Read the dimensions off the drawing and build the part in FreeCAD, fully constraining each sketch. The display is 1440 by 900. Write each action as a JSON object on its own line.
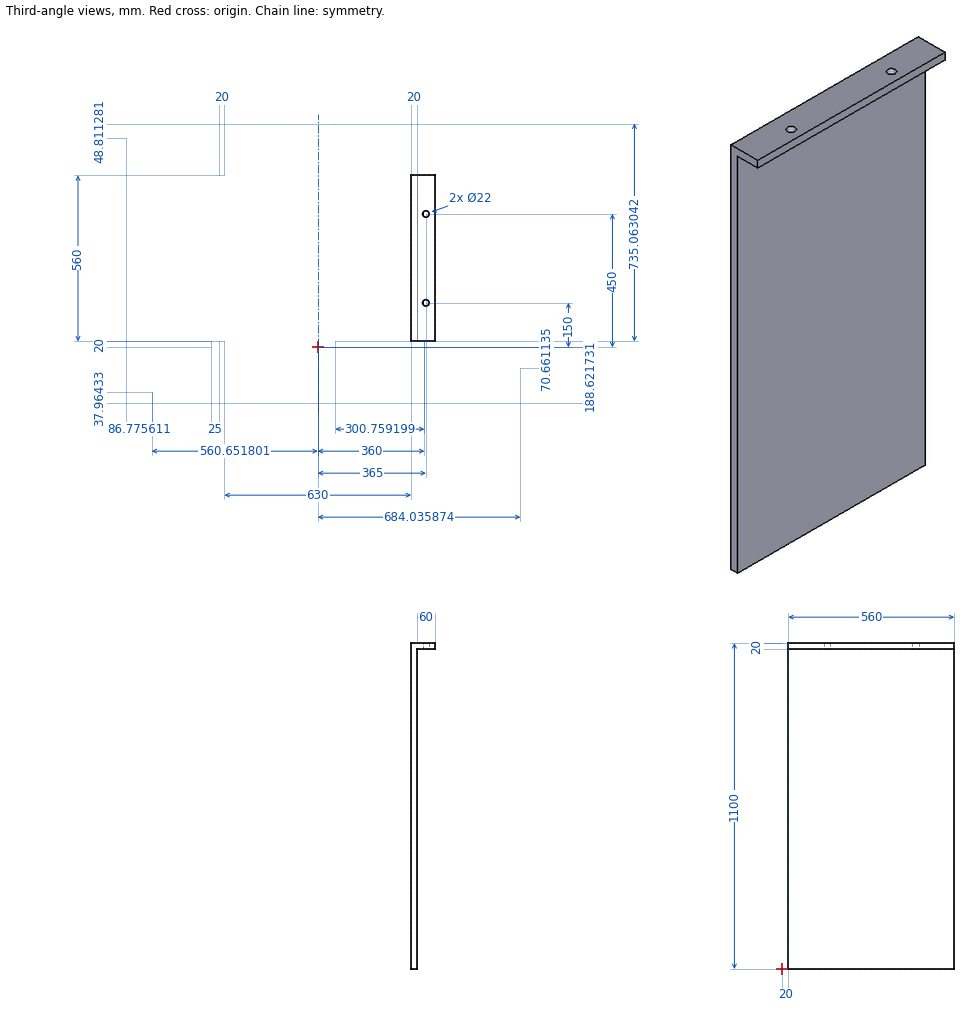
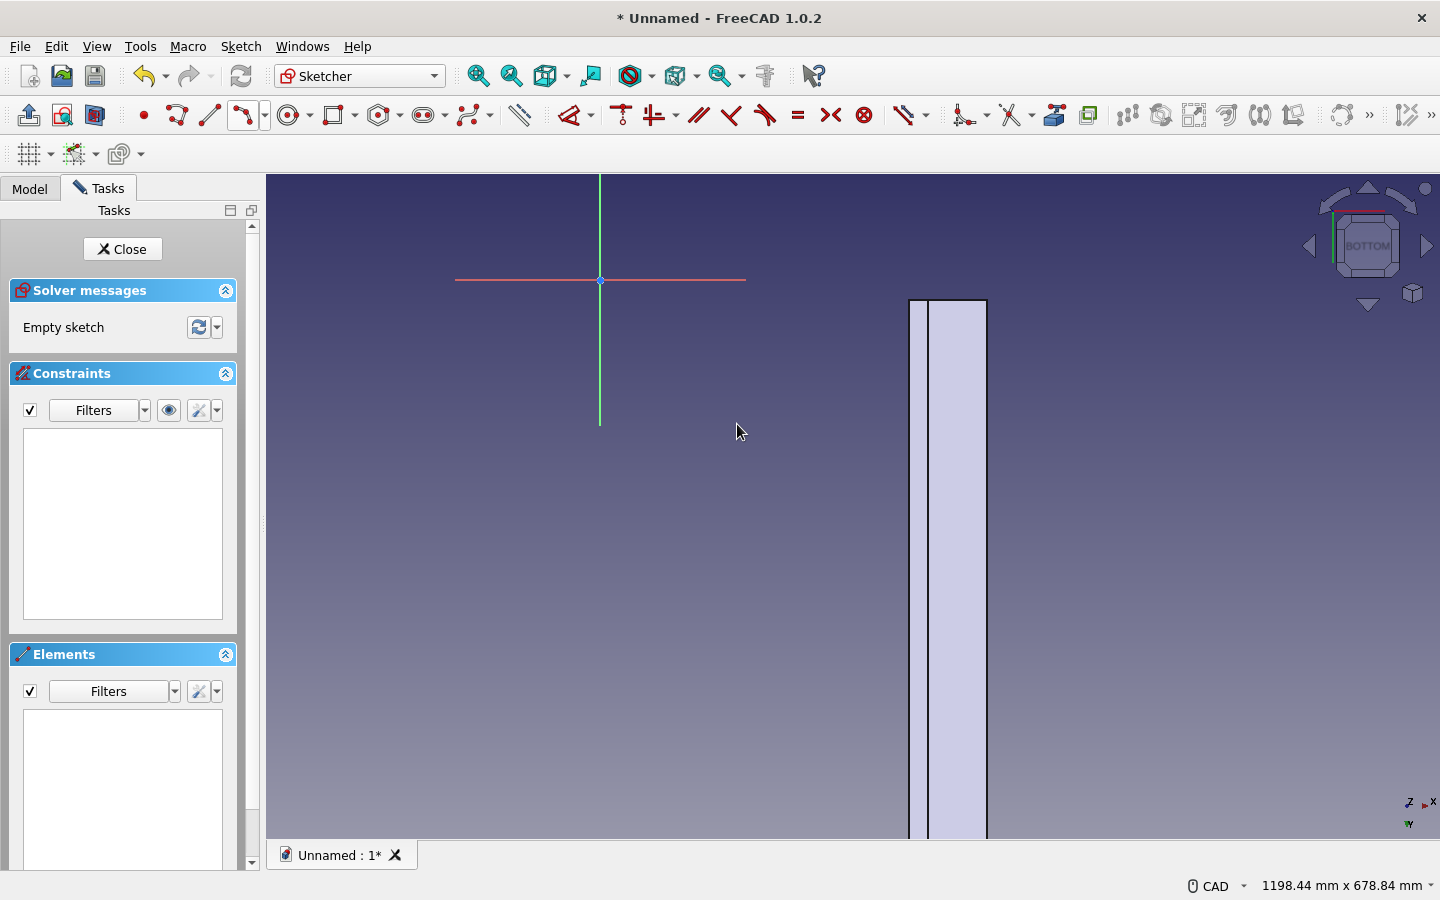
{"action": "key", "text": "g c"}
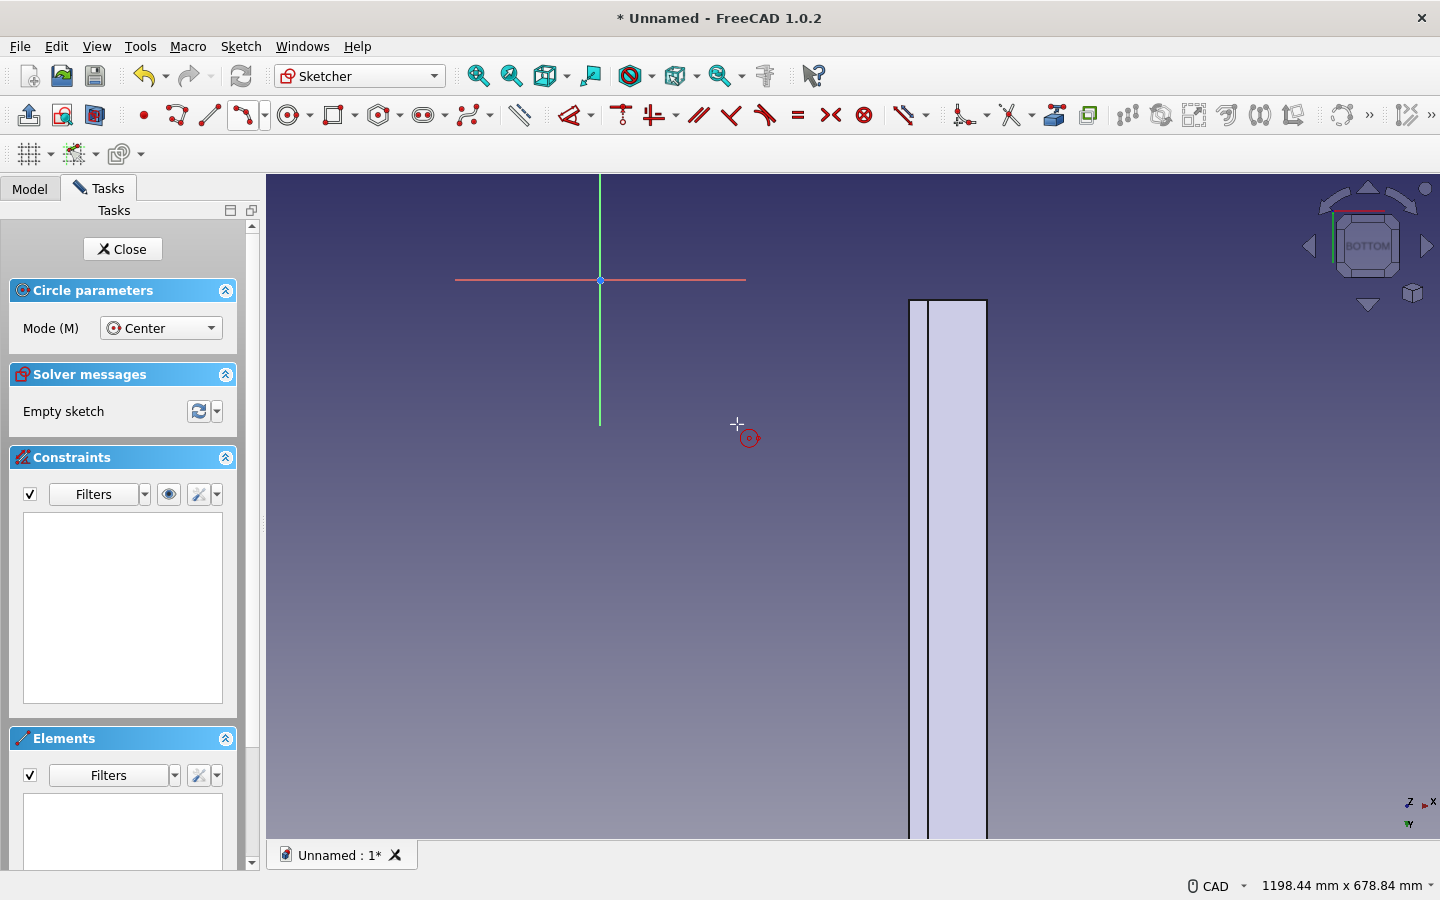
{"action": "scroll", "coordinate": [958, 721], "scroll_direction": "up", "scroll_amount": 4}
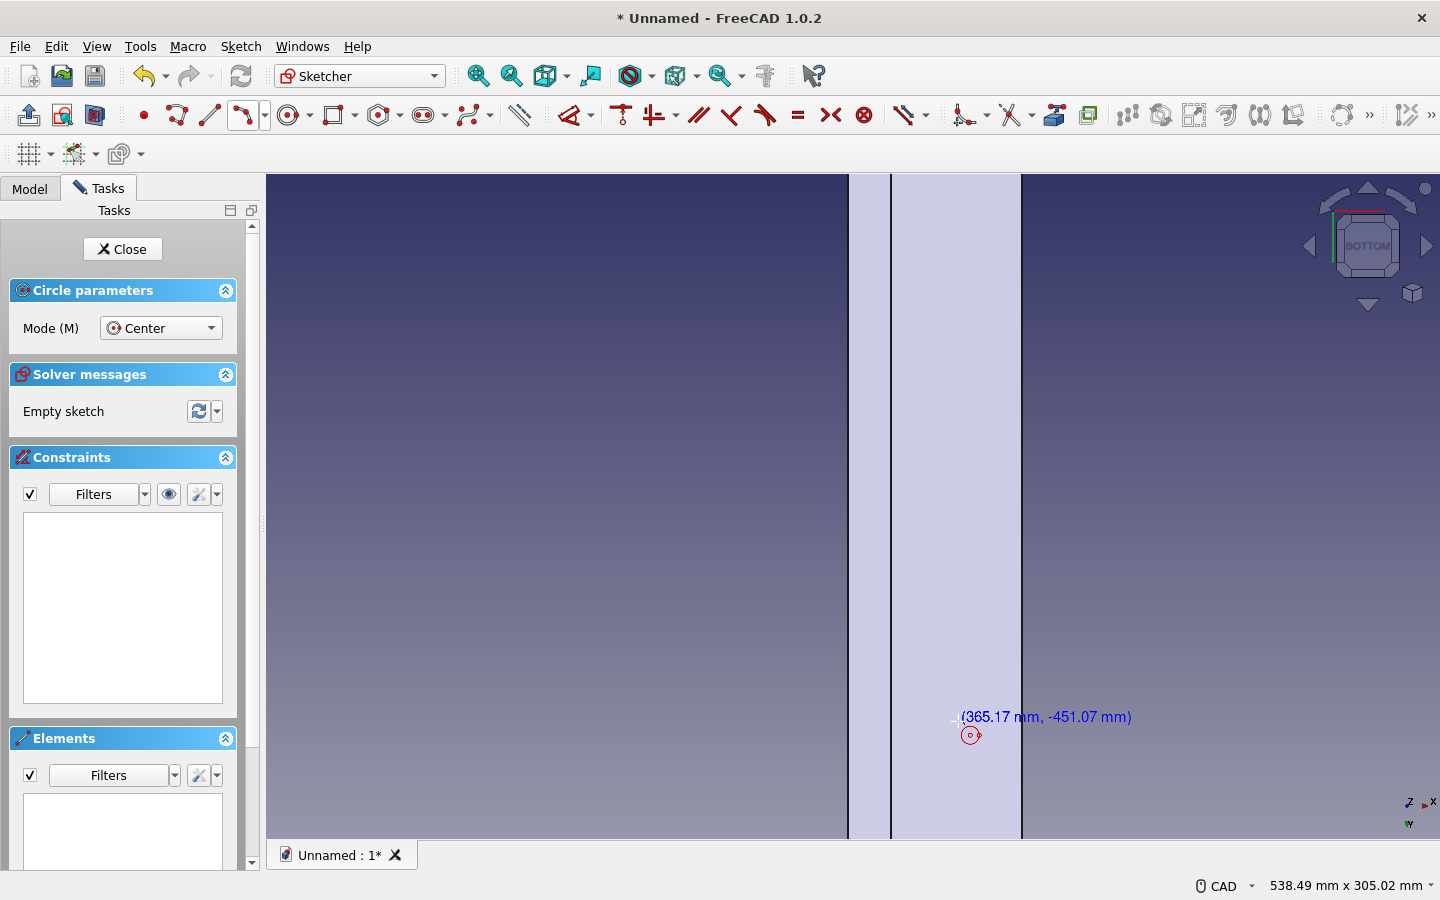
{"action": "left_click", "coordinate": [957, 720]}
{"action": "left_click", "coordinate": [974, 703]}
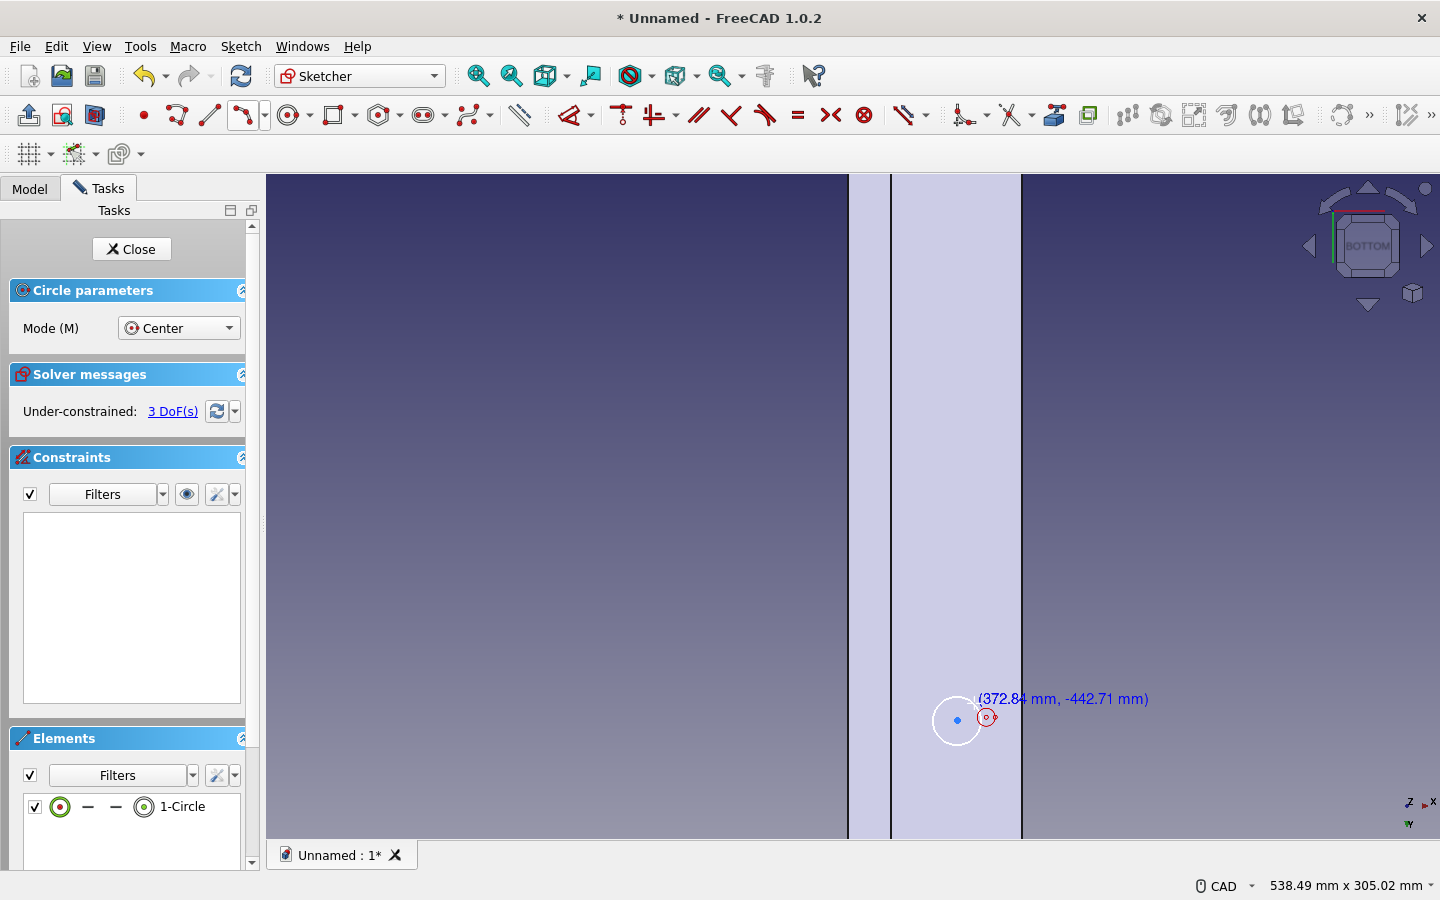
{"action": "scroll", "coordinate": [959, 723], "scroll_direction": "down", "scroll_amount": 4}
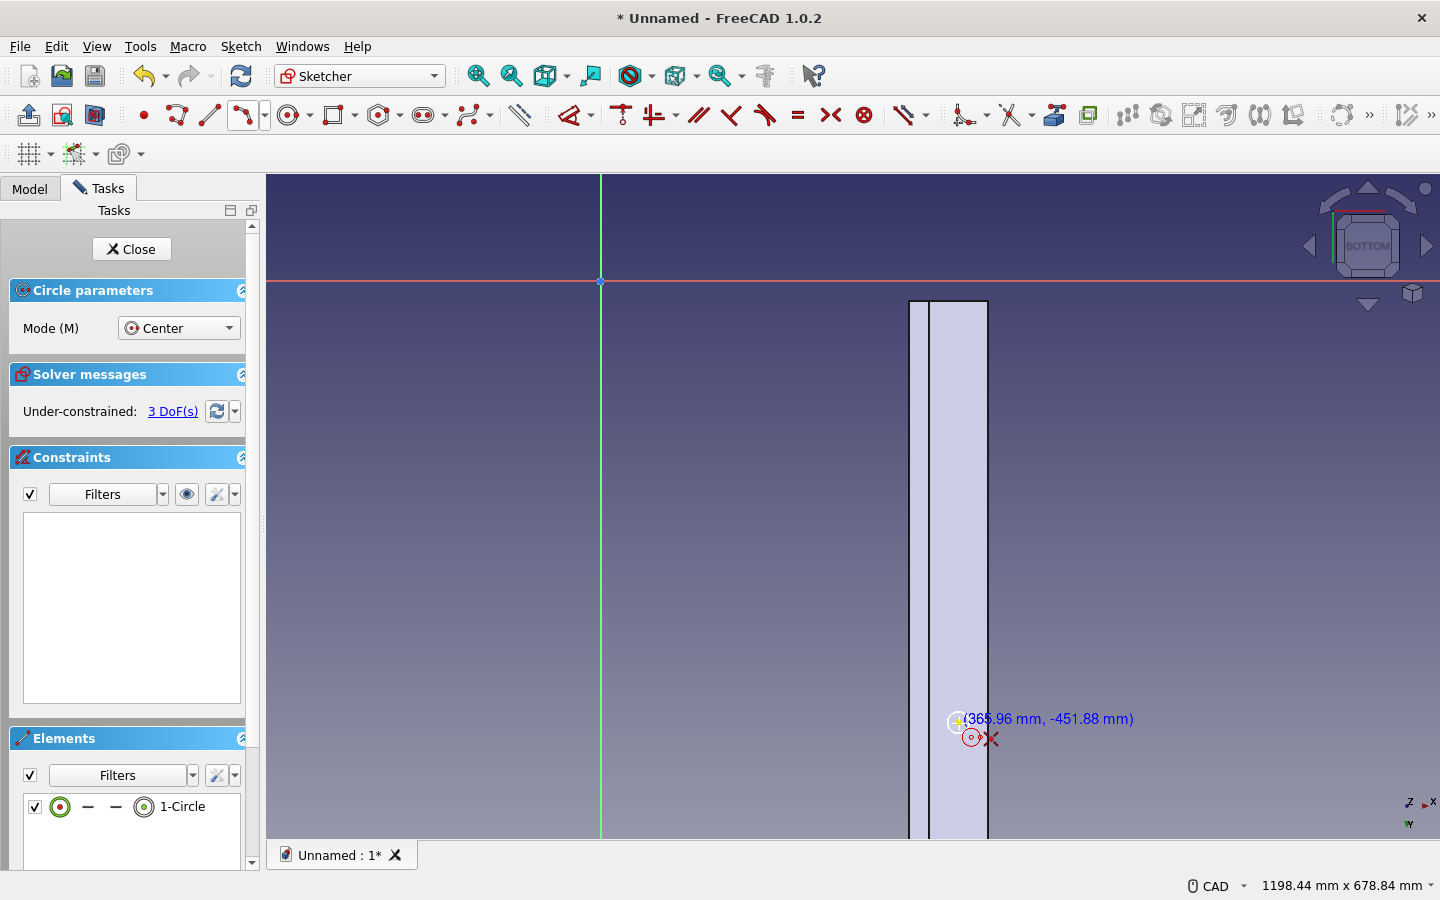
{"action": "scroll", "coordinate": [958, 428], "scroll_direction": "up", "scroll_amount": 4}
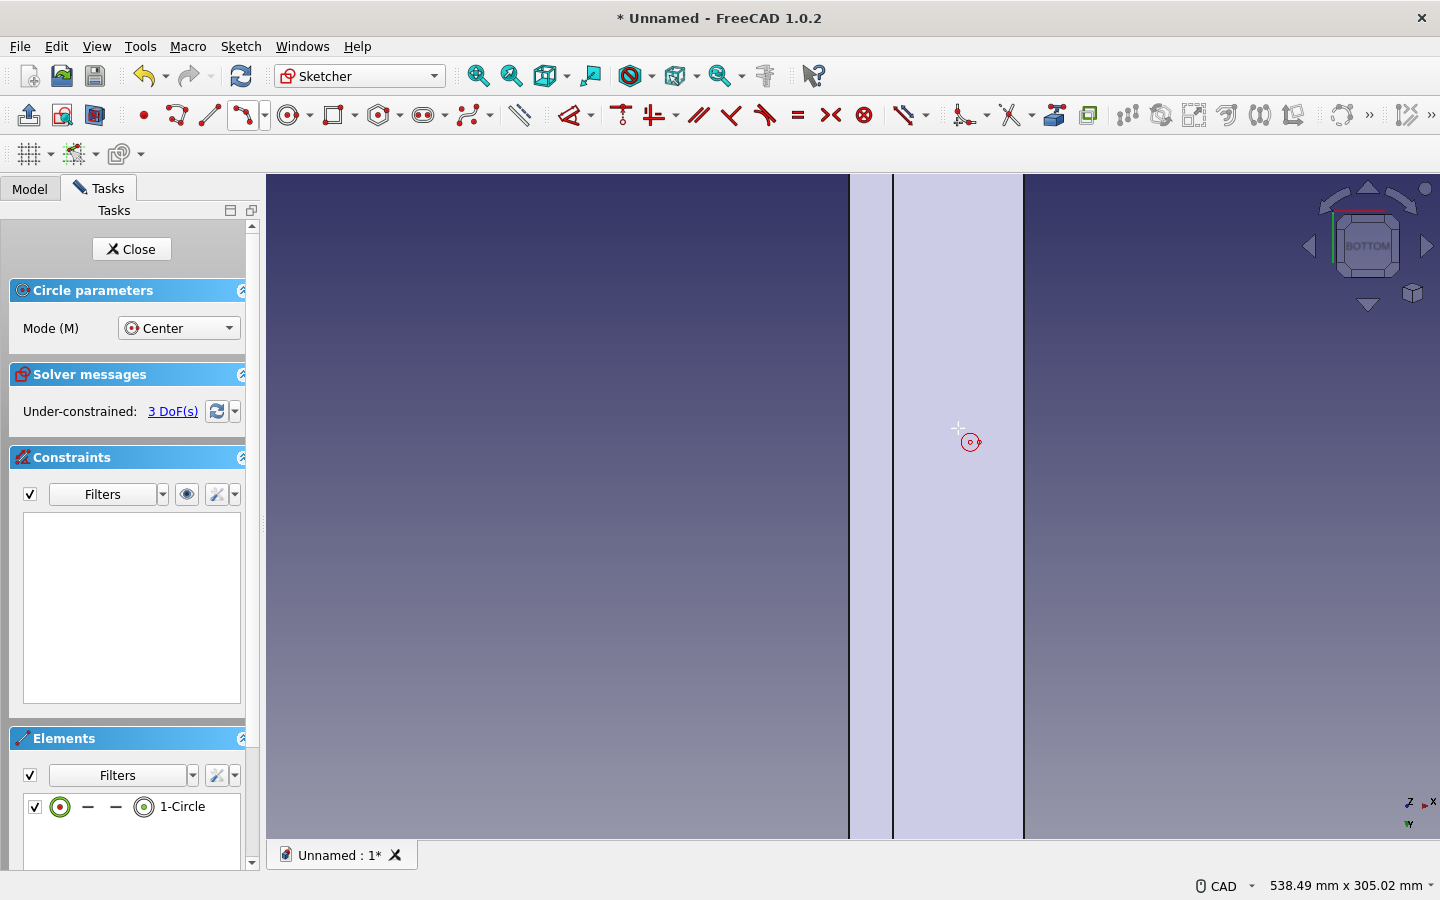
{"action": "left_click", "coordinate": [958, 428]}
{"action": "left_click", "coordinate": [975, 411]}
{"action": "key", "text": "Escape"}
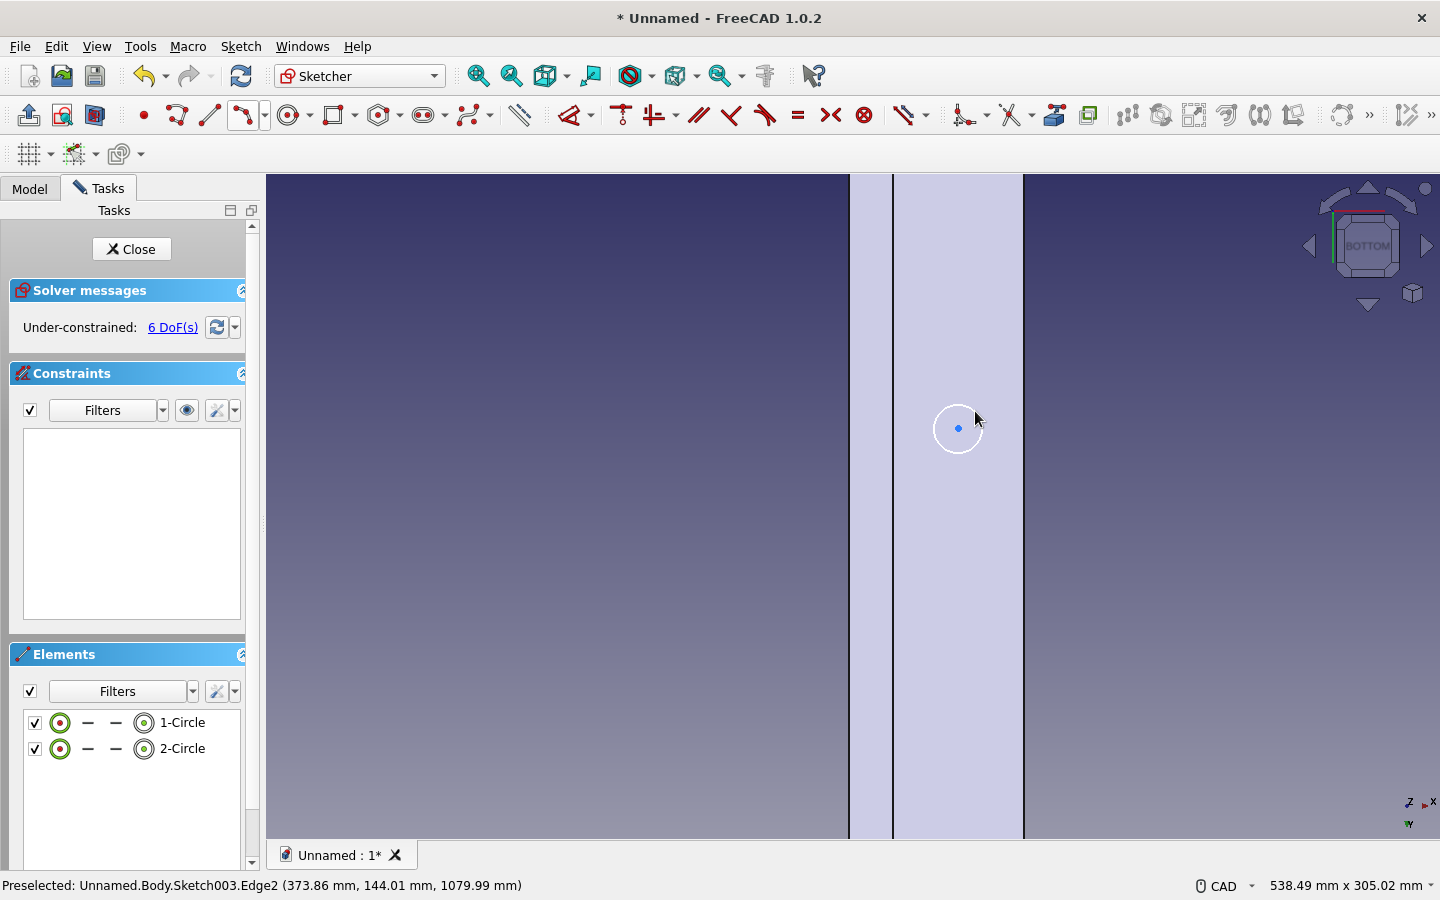
{"action": "scroll", "coordinate": [958, 427], "scroll_direction": "down", "scroll_amount": 4}